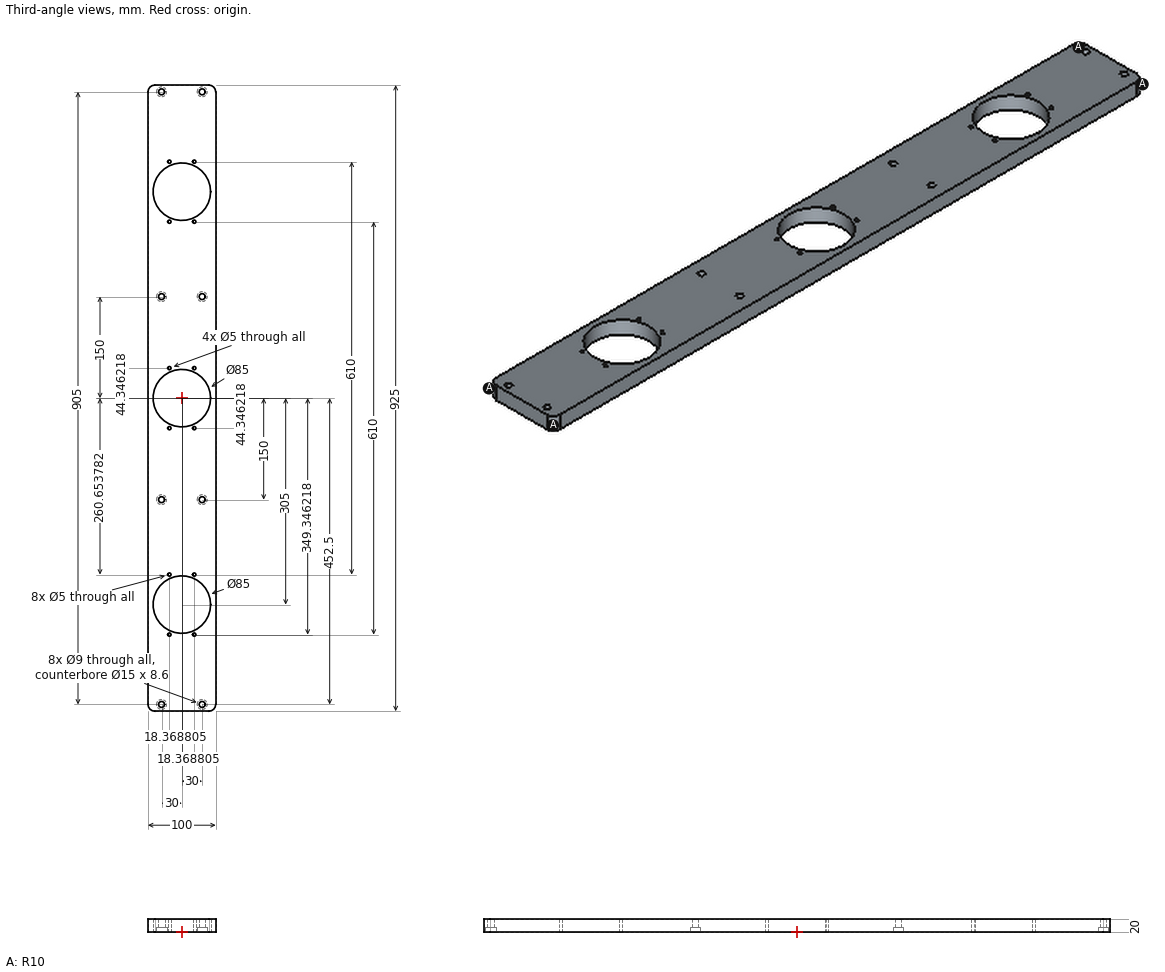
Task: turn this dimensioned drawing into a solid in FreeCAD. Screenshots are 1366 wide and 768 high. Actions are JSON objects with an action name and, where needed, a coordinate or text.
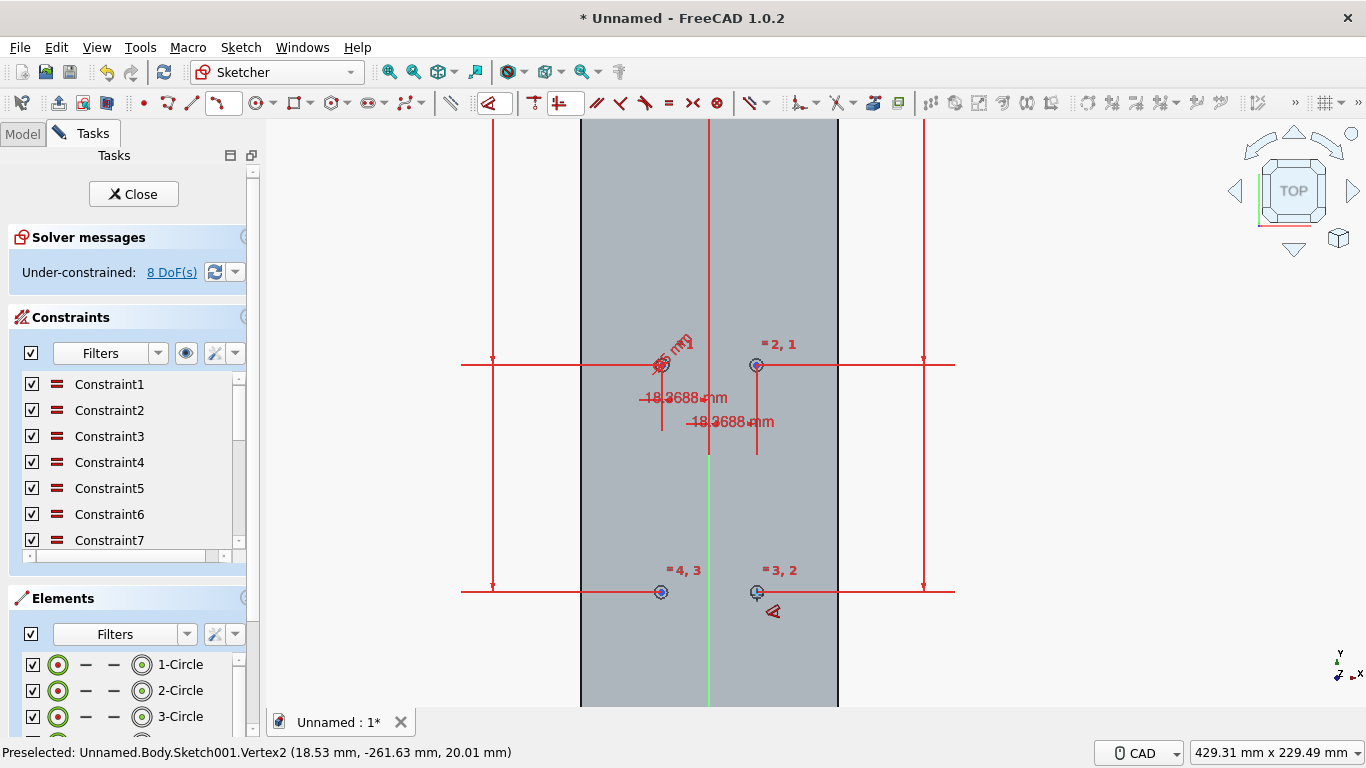
{"action": "left_click", "coordinate": [757, 592]}
{"action": "left_click", "coordinate": [733, 626]}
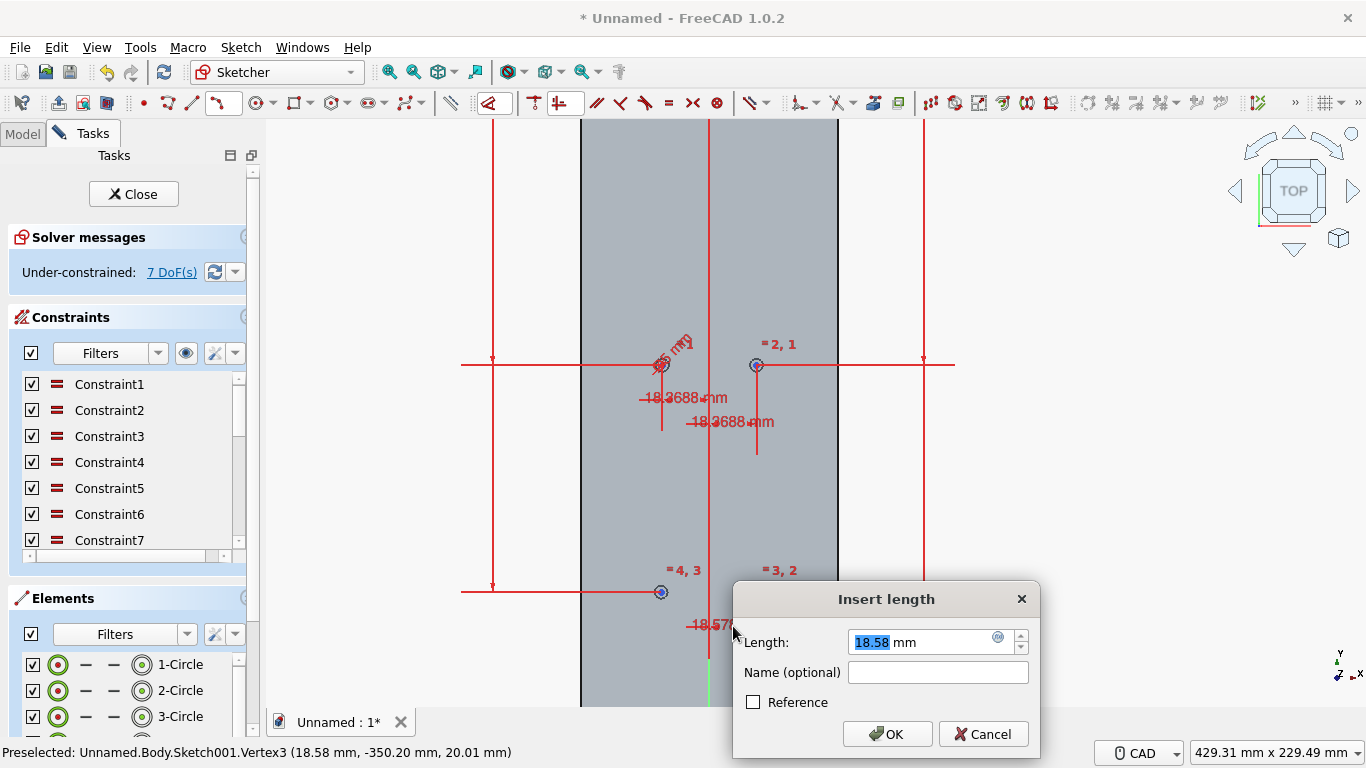
{"action": "type", "text": "18.368805"}
{"action": "key", "text": "Return"}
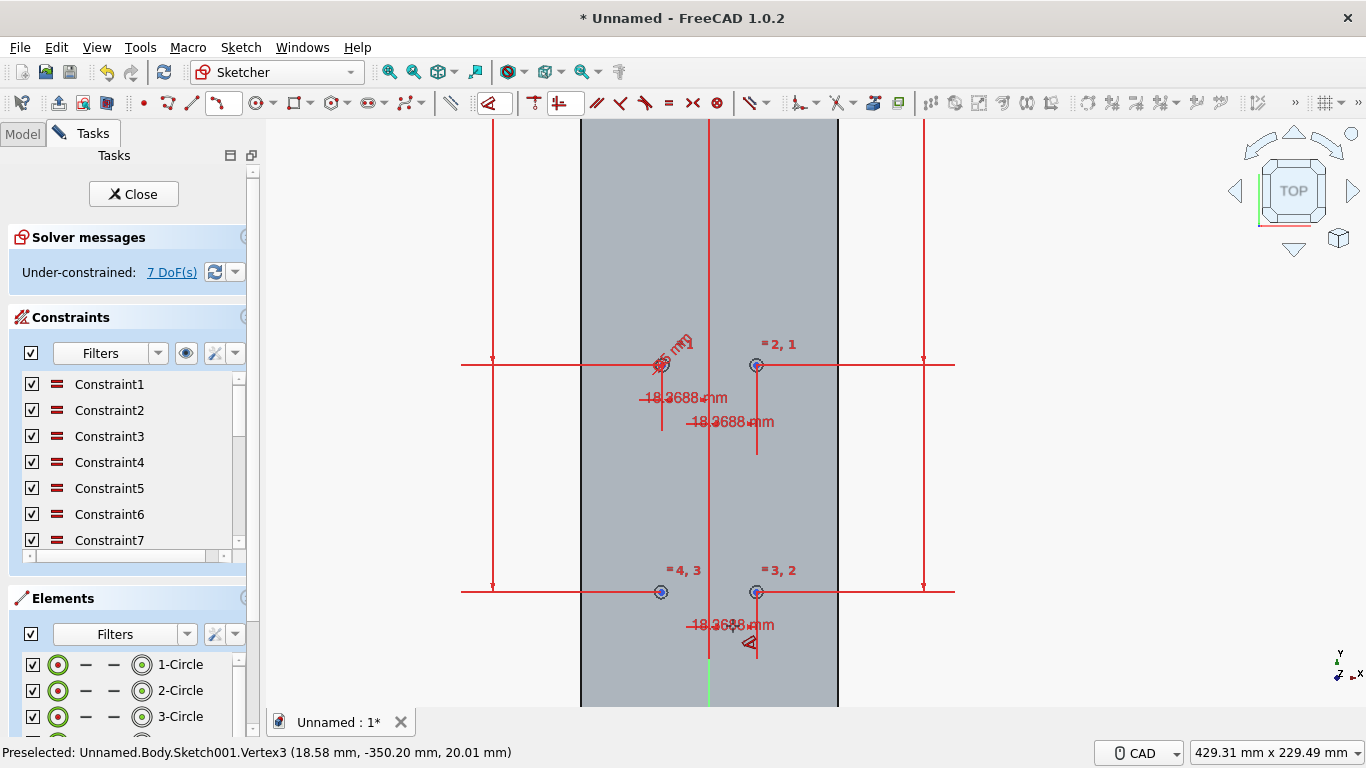
{"action": "left_click", "coordinate": [661, 592]}
{"action": "left_click", "coordinate": [685, 650]}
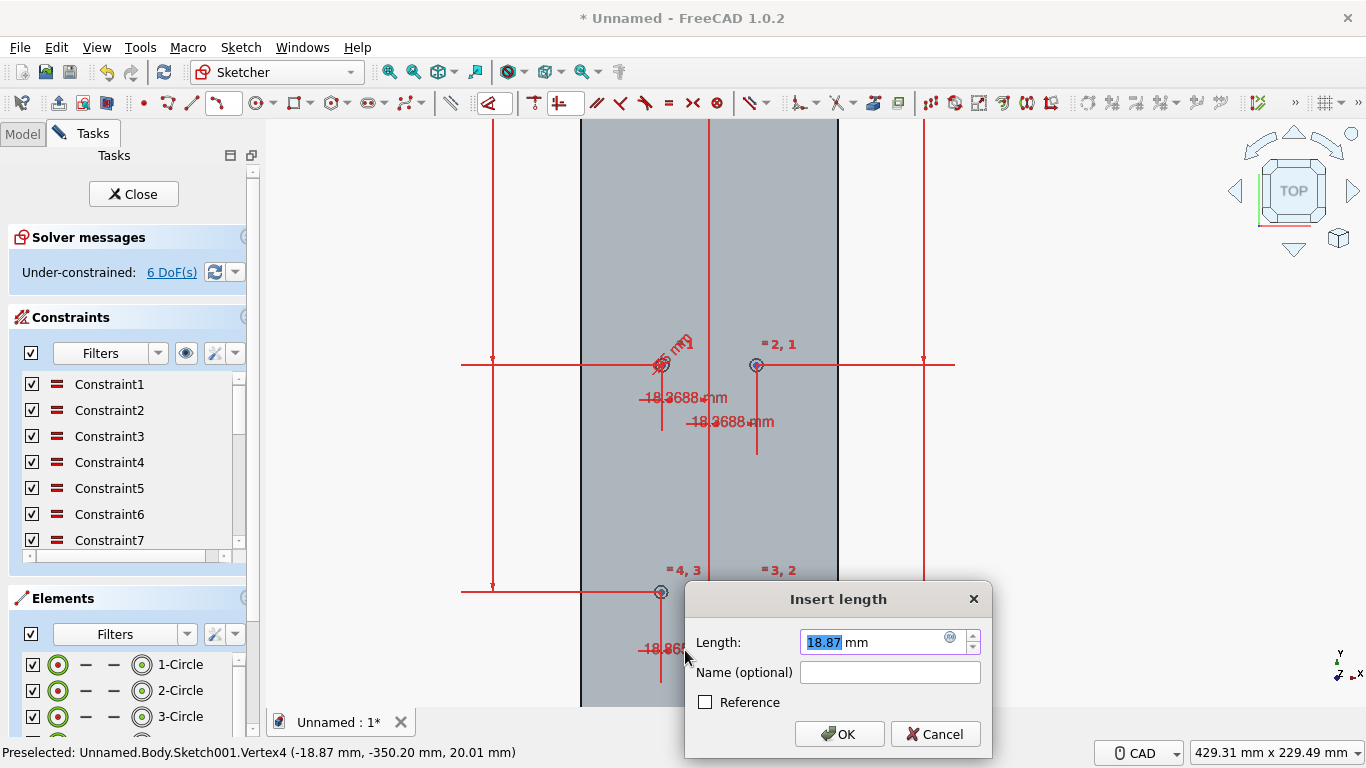
{"action": "type", "text": "18.368805"}
{"action": "key", "text": "Return"}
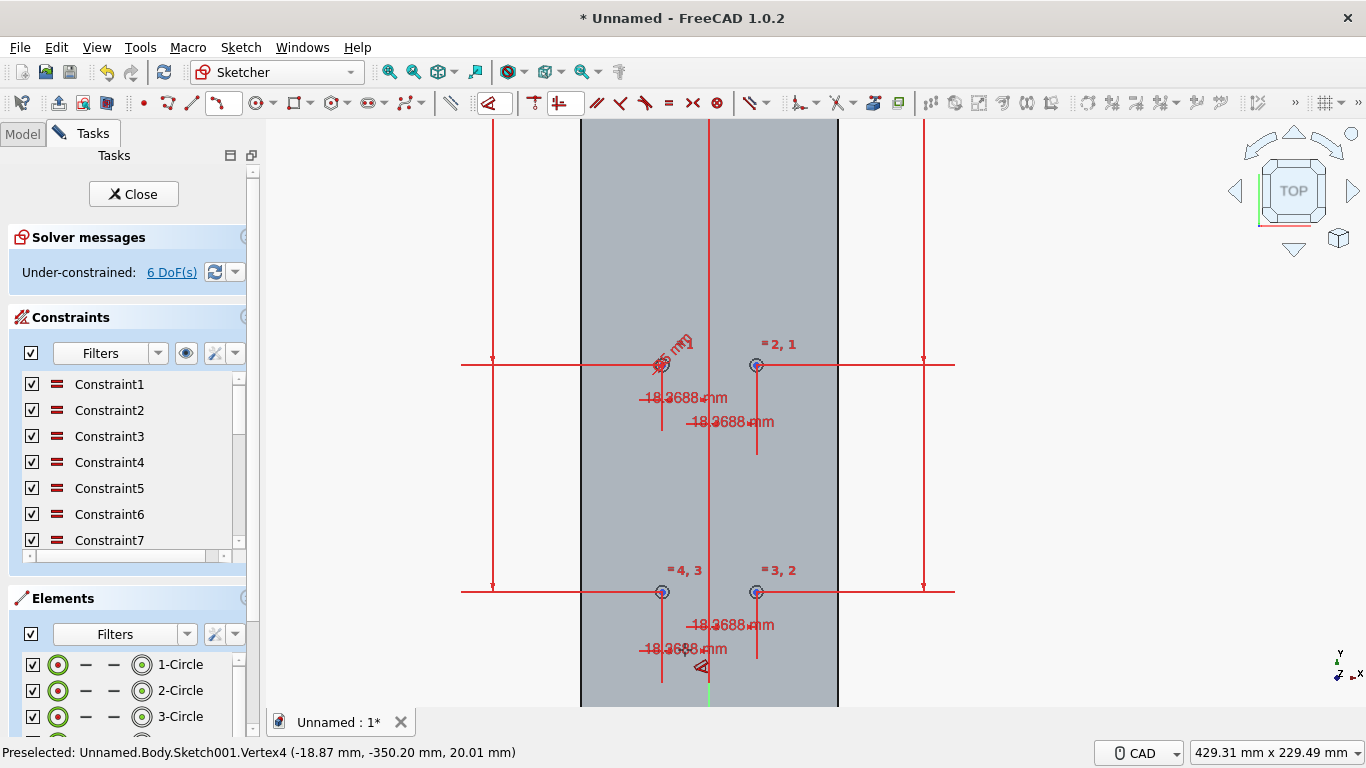
{"action": "scroll", "coordinate": [757, 595], "scroll_direction": "down", "scroll_amount": 8}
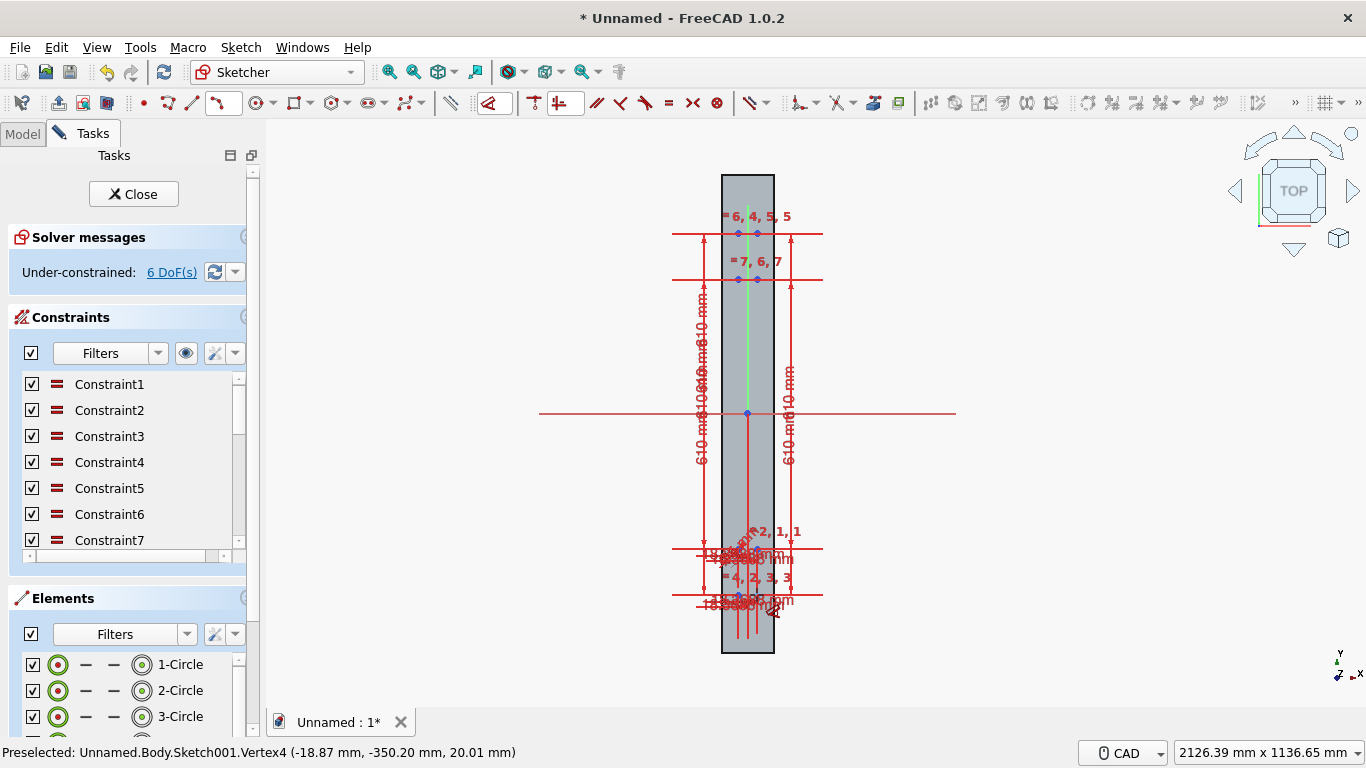
{"action": "scroll", "coordinate": [757, 234], "scroll_direction": "up", "scroll_amount": 8}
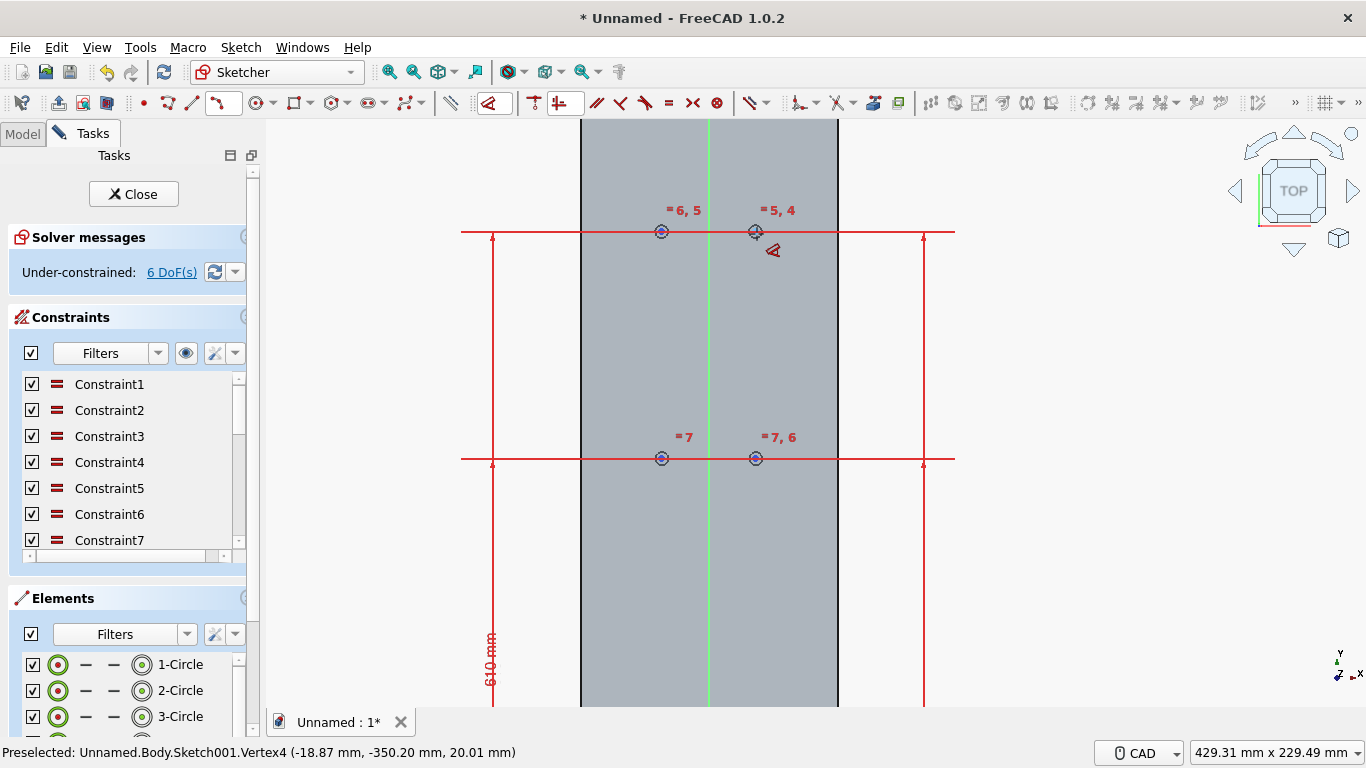
{"action": "left_click", "coordinate": [755, 232]}
{"action": "left_click", "coordinate": [732, 198]}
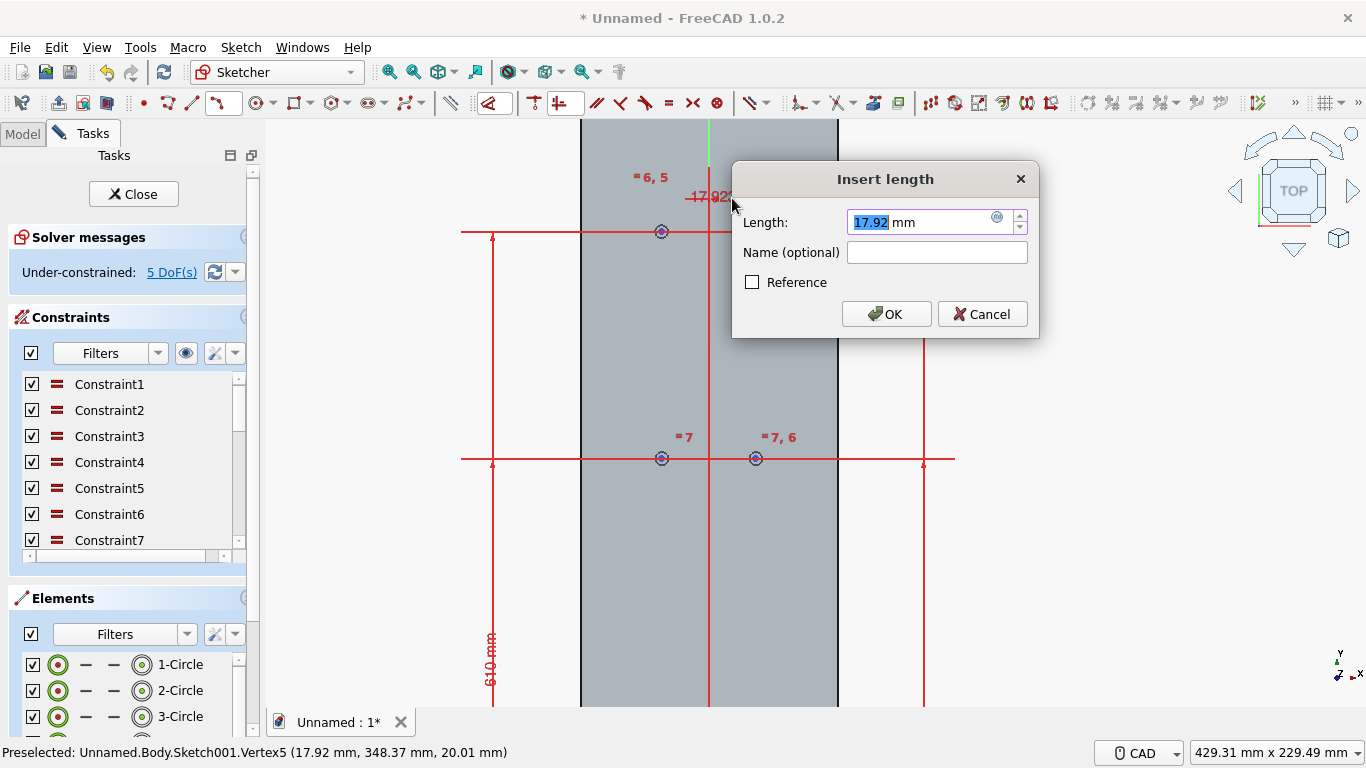
{"action": "type", "text": "18.368805"}
{"action": "key", "text": "Return"}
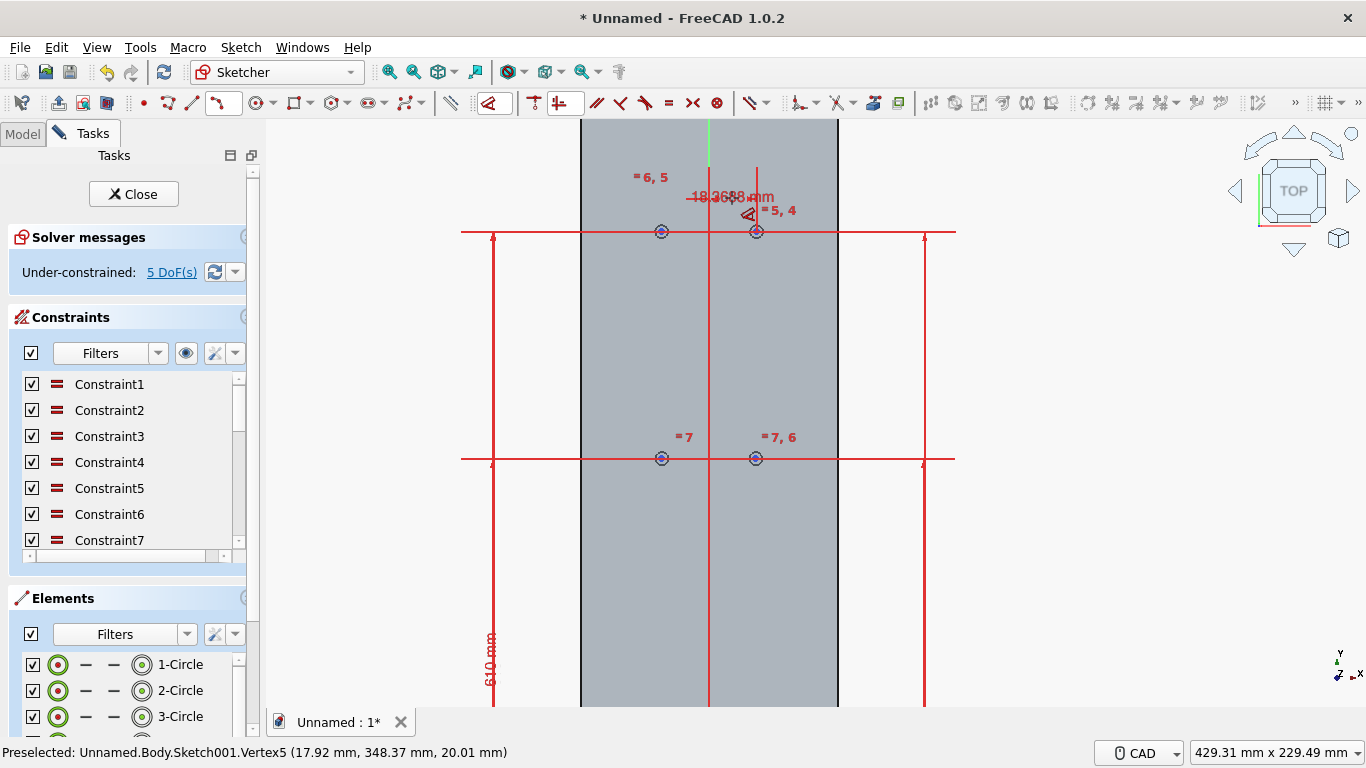
{"action": "left_click", "coordinate": [662, 232]}
{"action": "left_click", "coordinate": [686, 174]}